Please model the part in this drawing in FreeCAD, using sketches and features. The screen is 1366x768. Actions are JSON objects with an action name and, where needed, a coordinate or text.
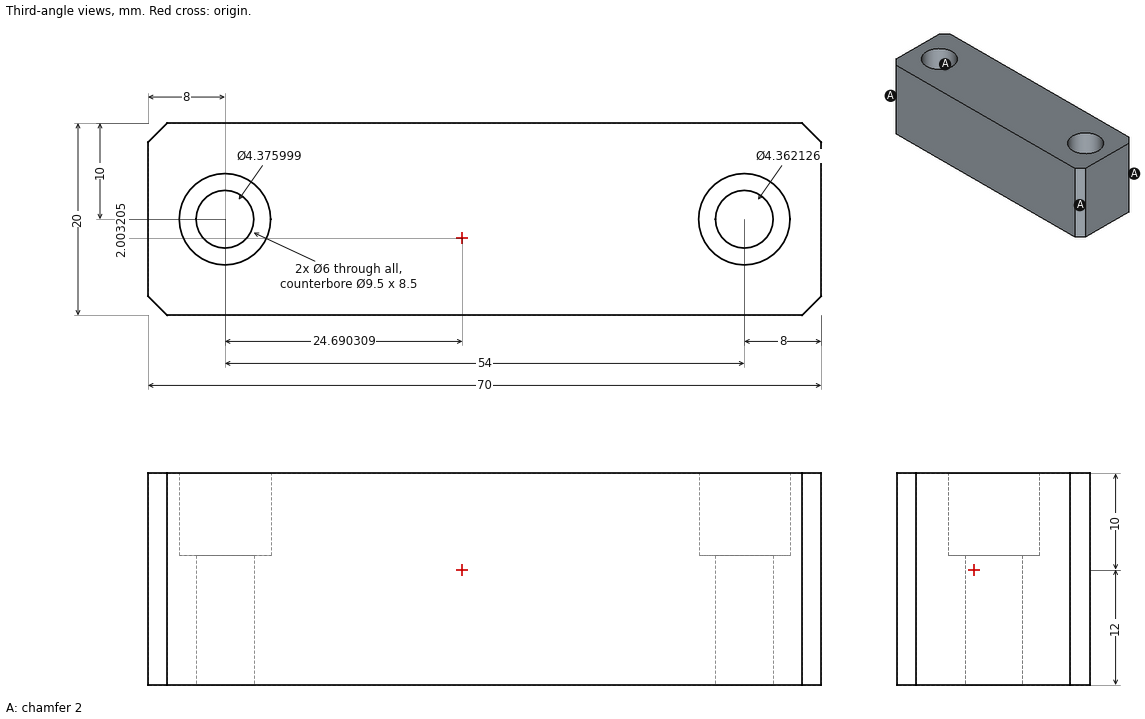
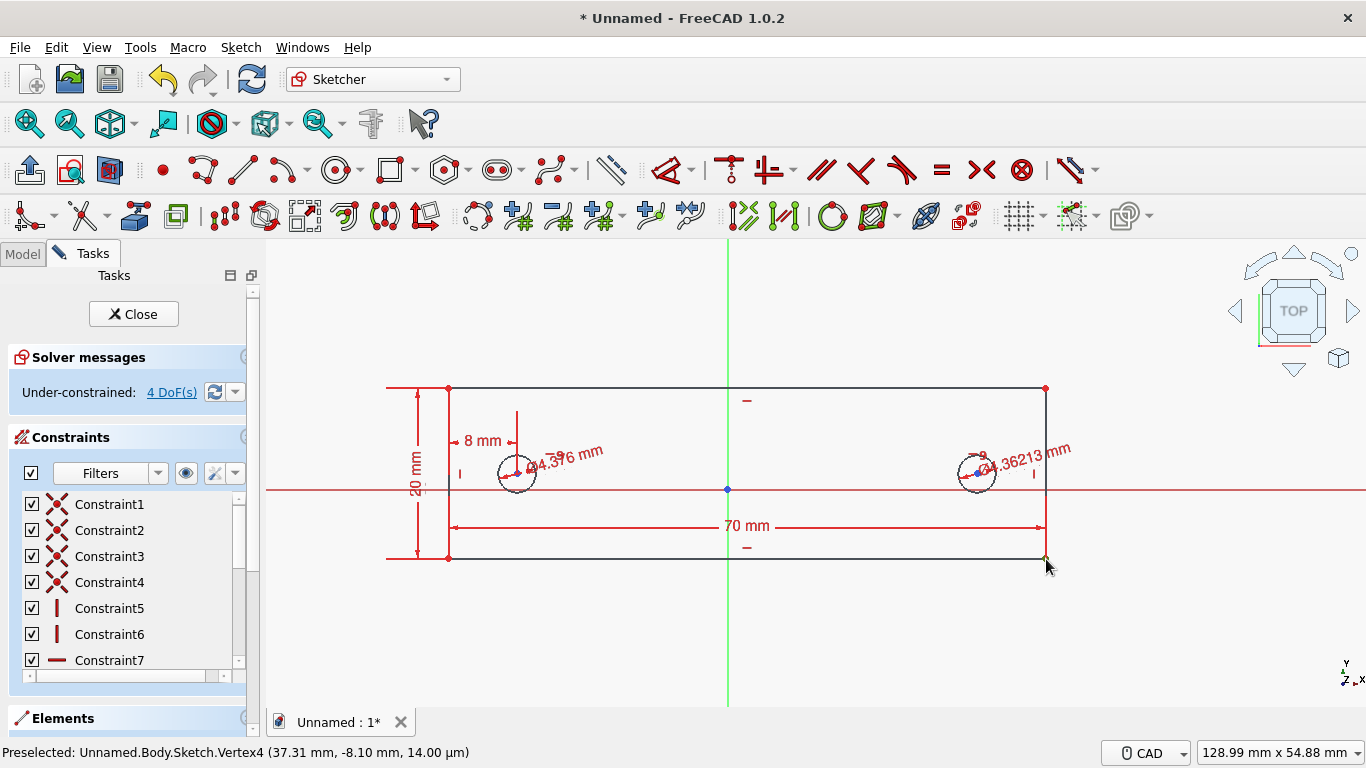
{"action": "left_click", "coordinate": [977, 474]}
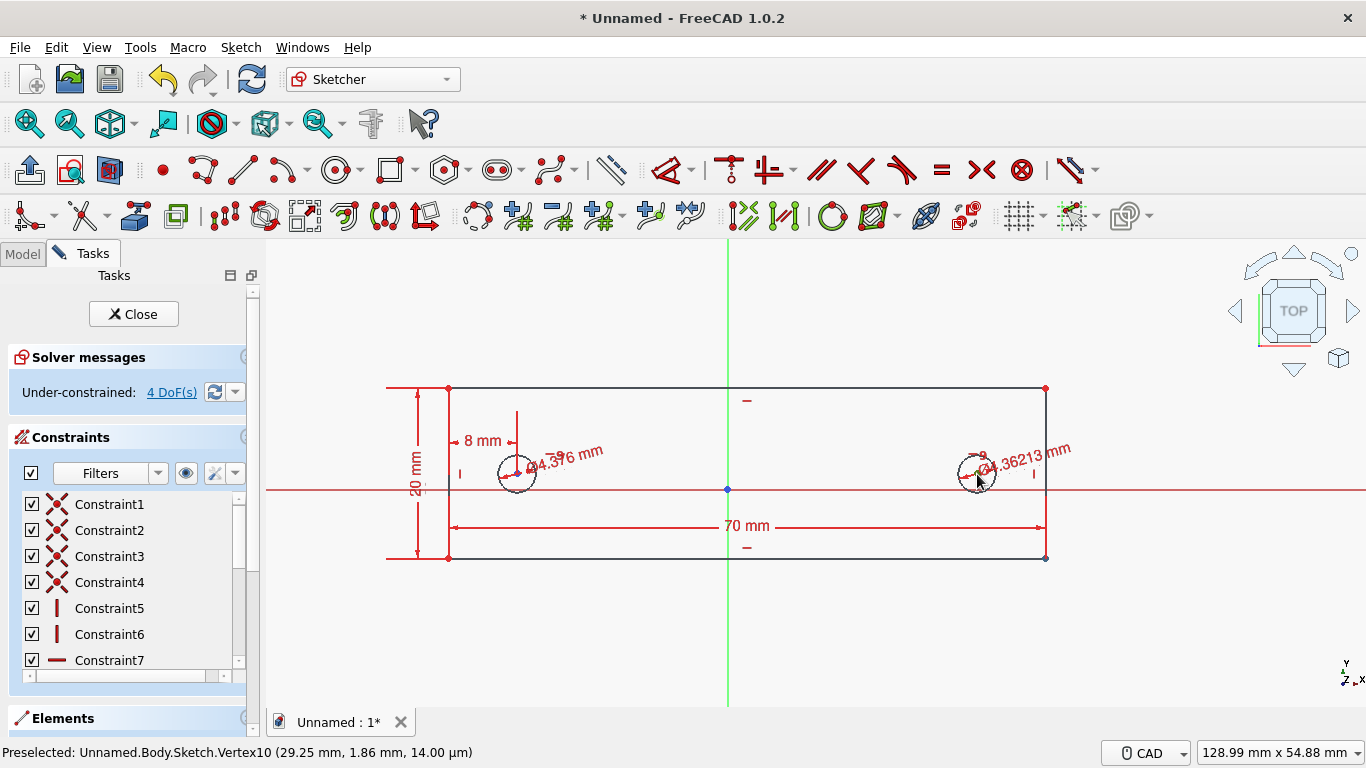
{"action": "left_click", "coordinate": [694, 170]}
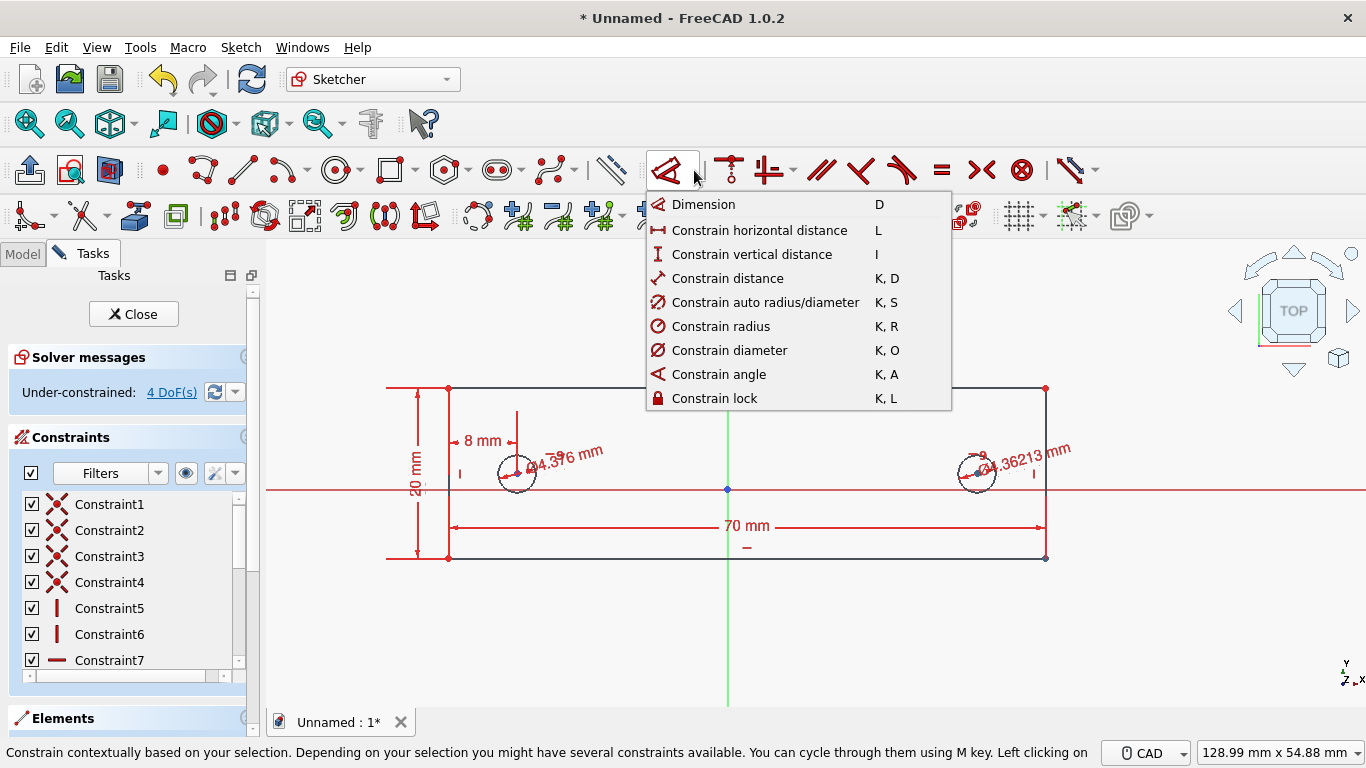
{"action": "left_click", "coordinate": [799, 230]}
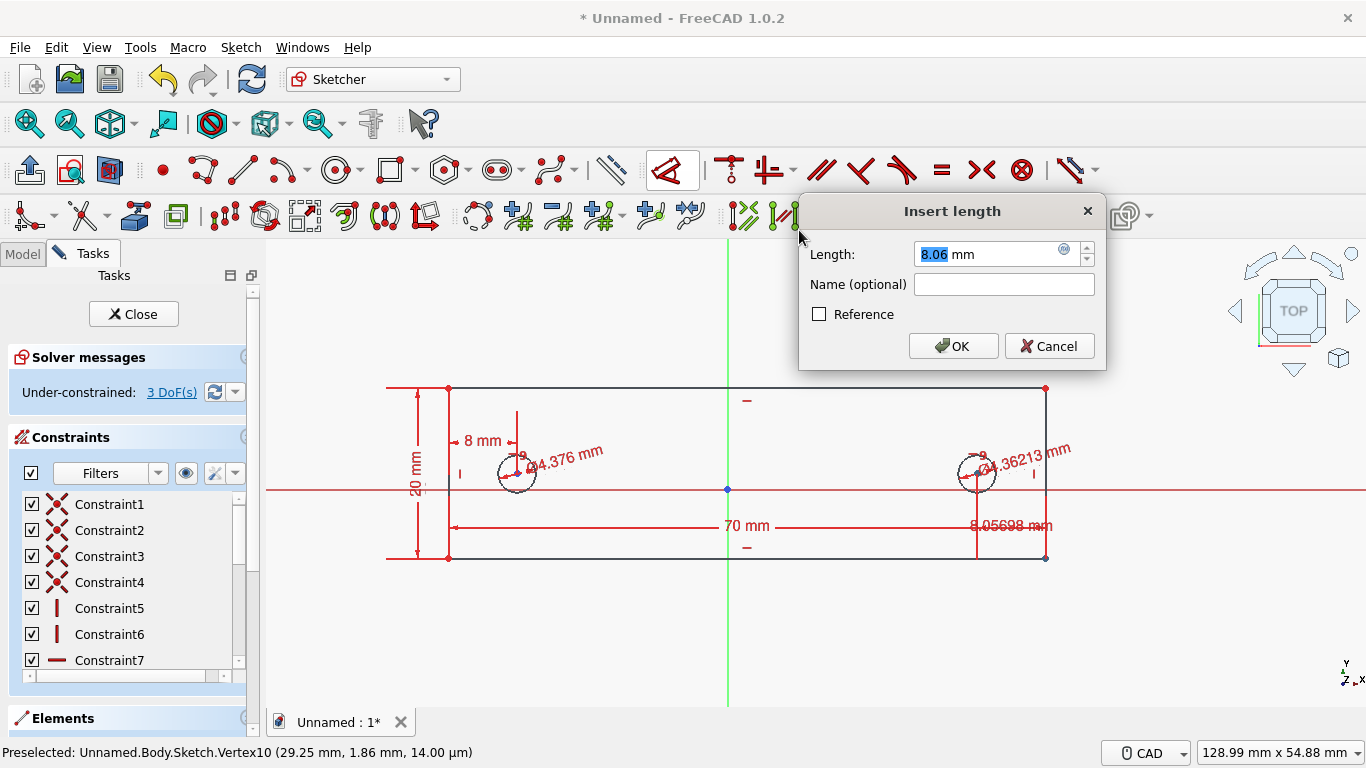
{"action": "type", "text": "8"}
{"action": "key", "text": "Return"}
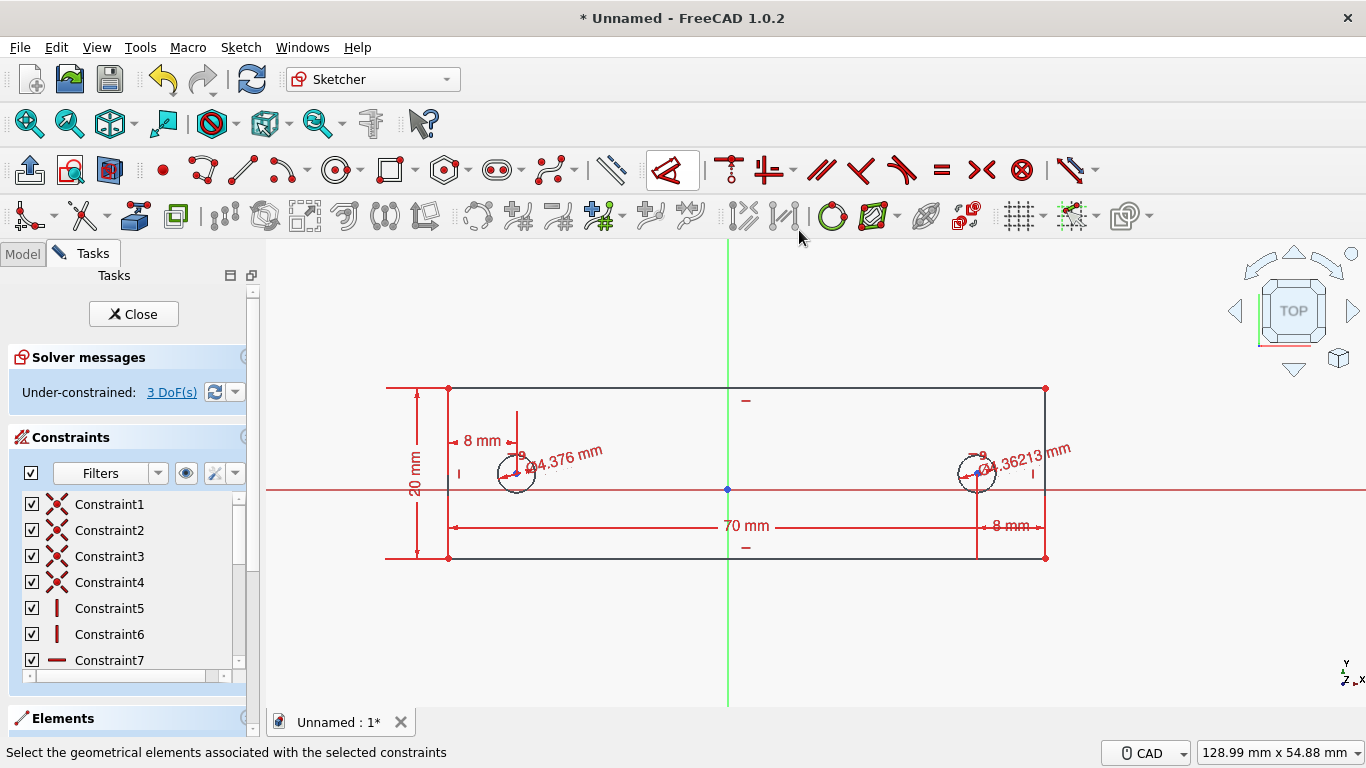
{"action": "left_click", "coordinate": [448, 388]}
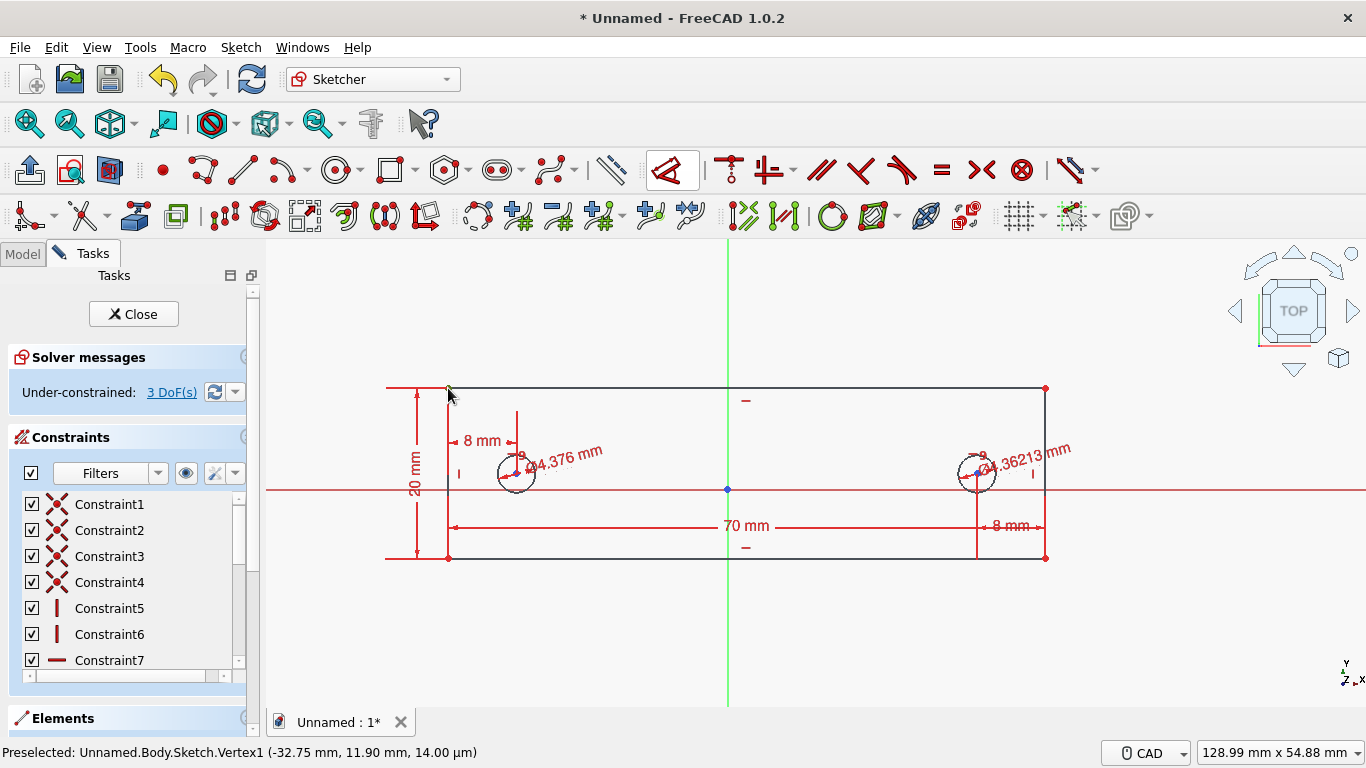
{"action": "left_click", "coordinate": [517, 474]}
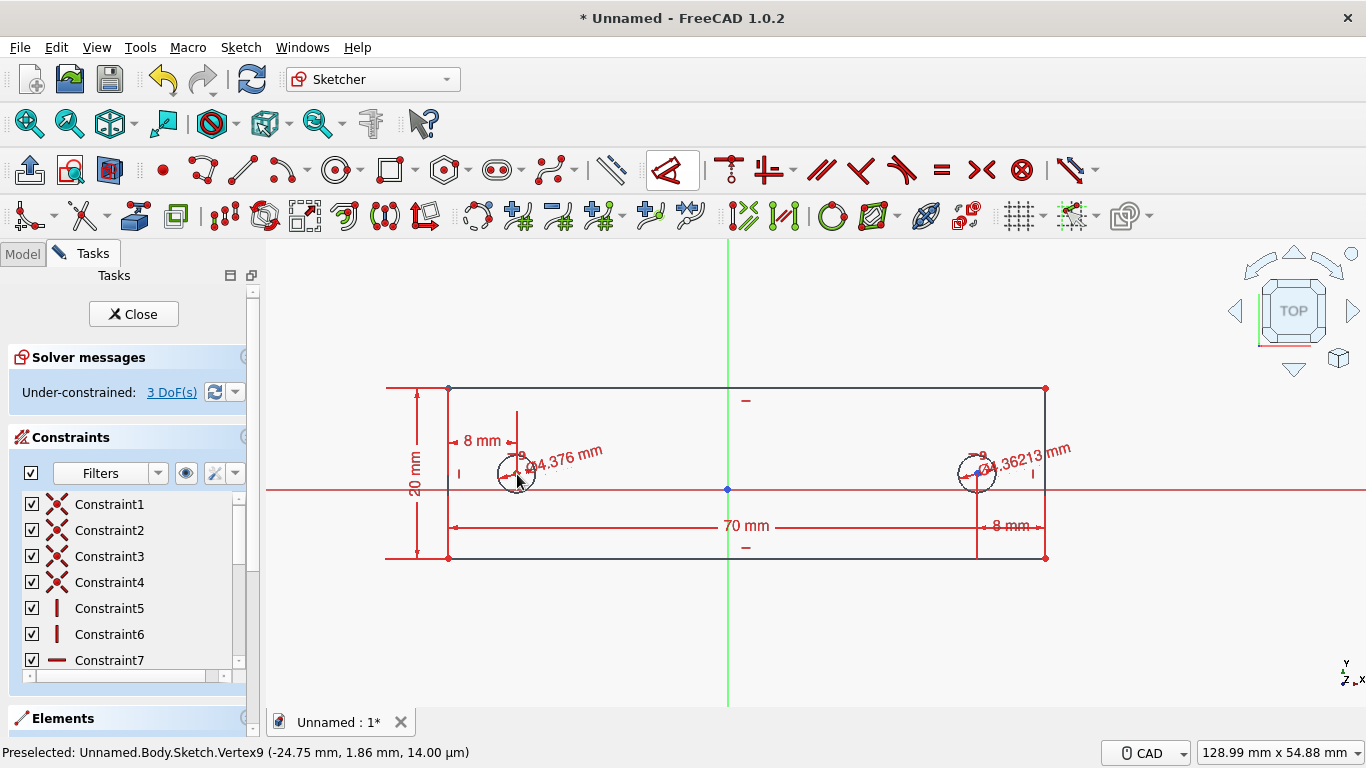
{"action": "key", "text": "i"}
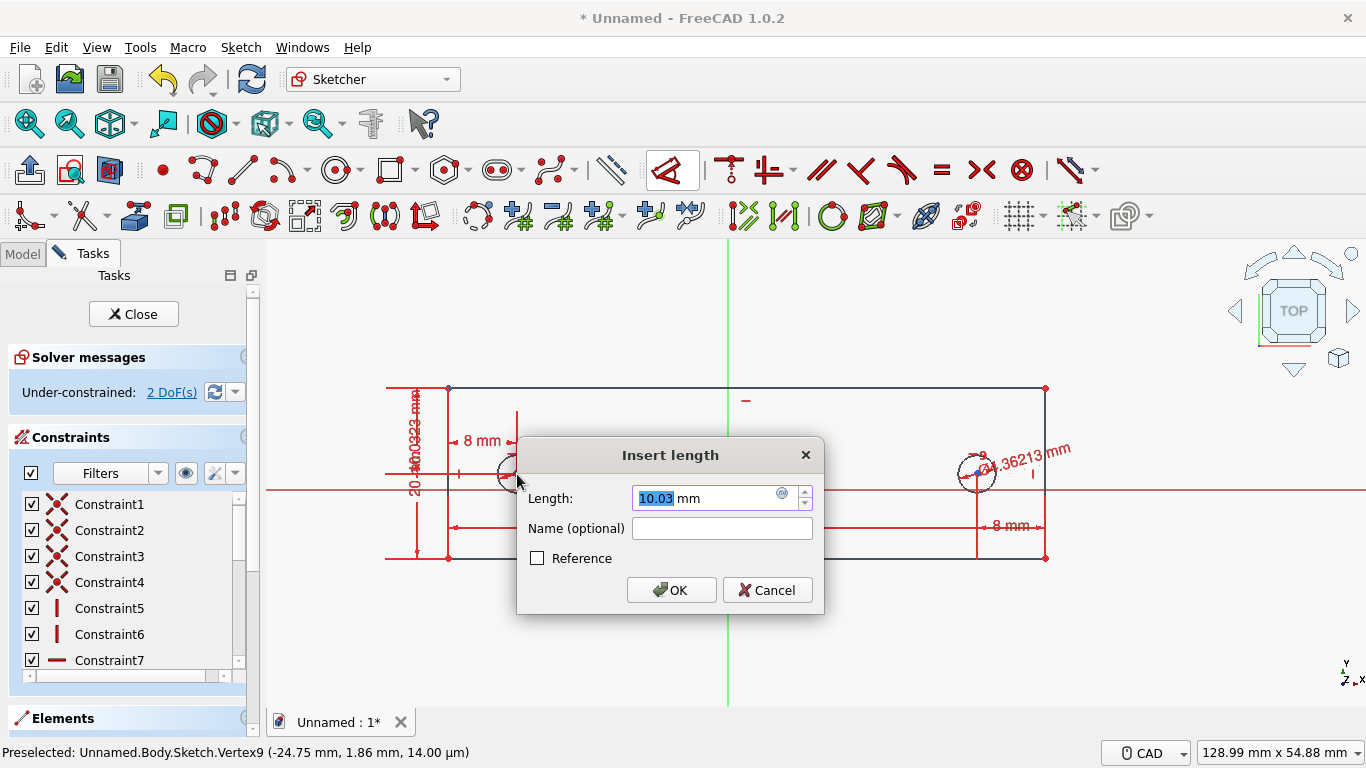
{"action": "type", "text": "10"}
{"action": "key", "text": "Return"}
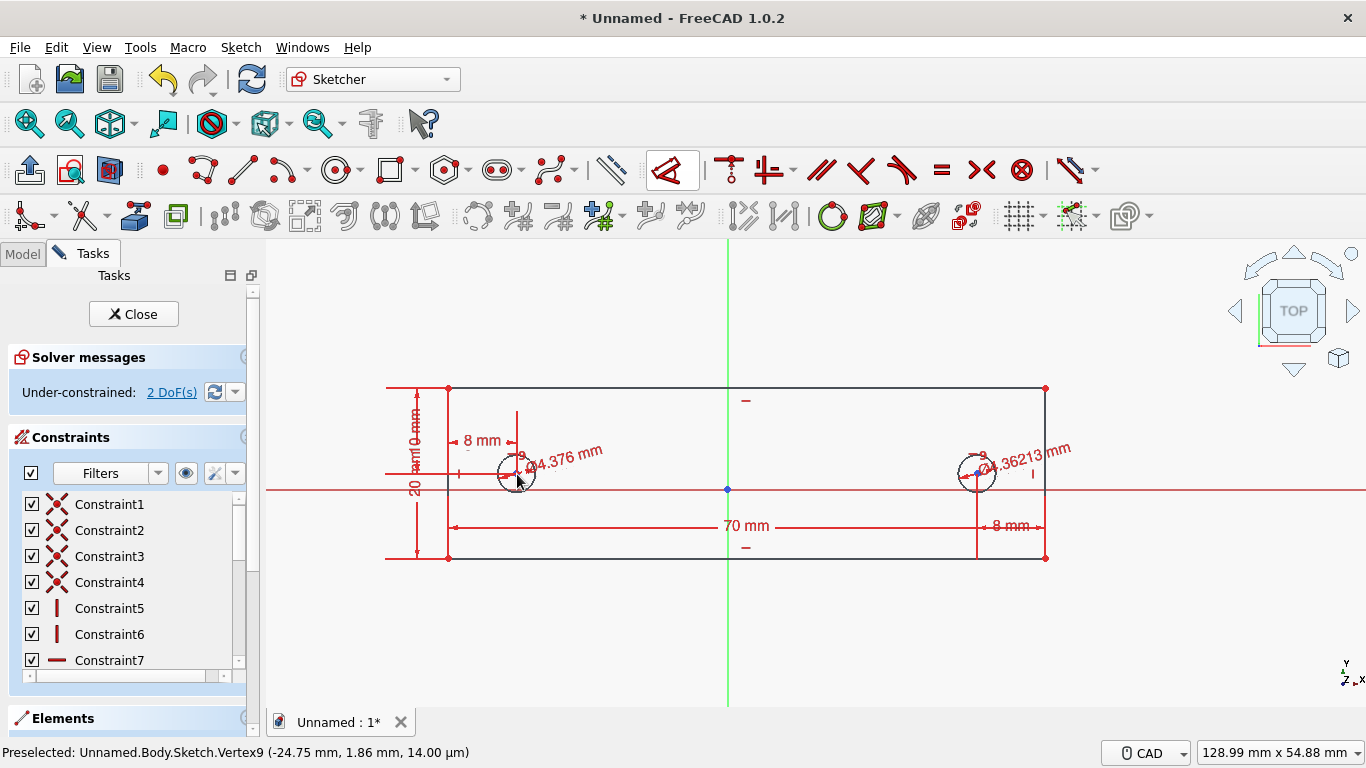
{"action": "scroll", "coordinate": [517, 474], "scroll_direction": "up", "scroll_amount": 5}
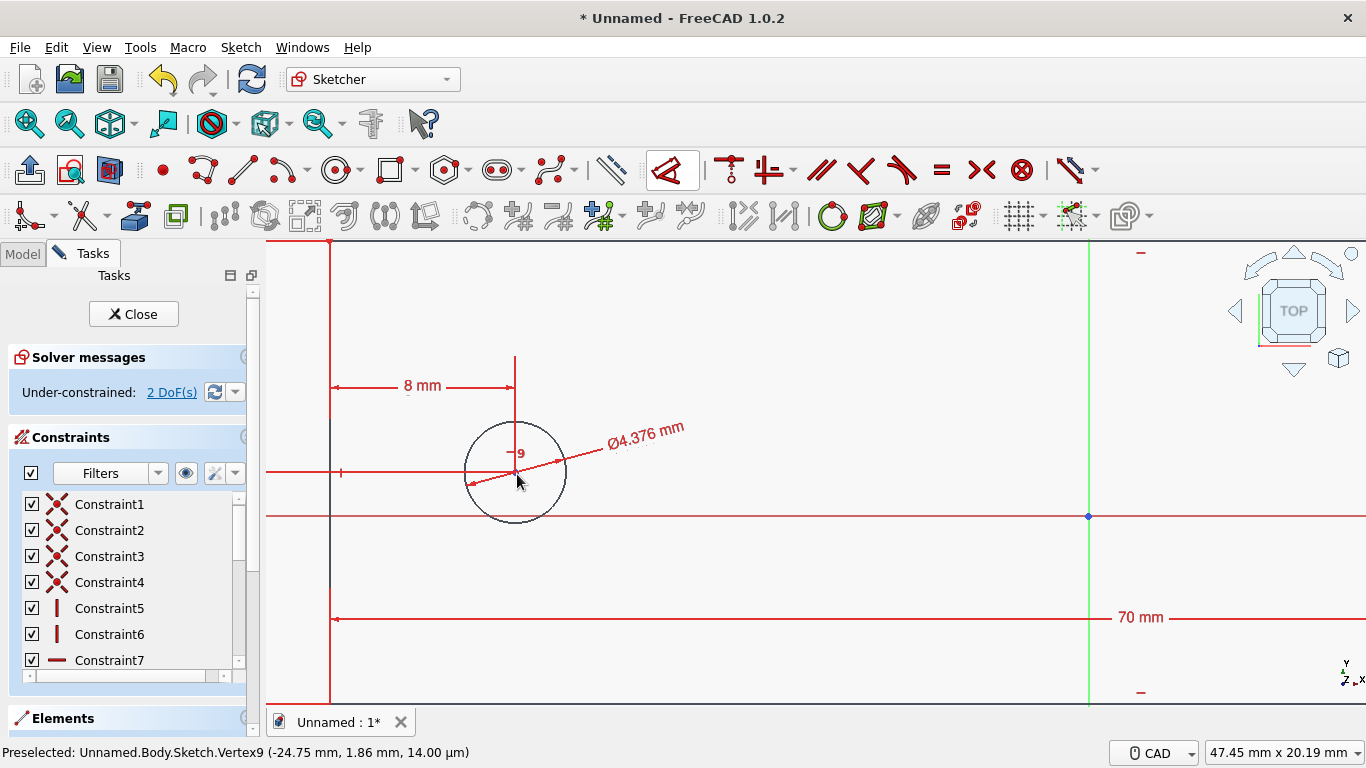
{"action": "left_click", "coordinate": [515, 472]}